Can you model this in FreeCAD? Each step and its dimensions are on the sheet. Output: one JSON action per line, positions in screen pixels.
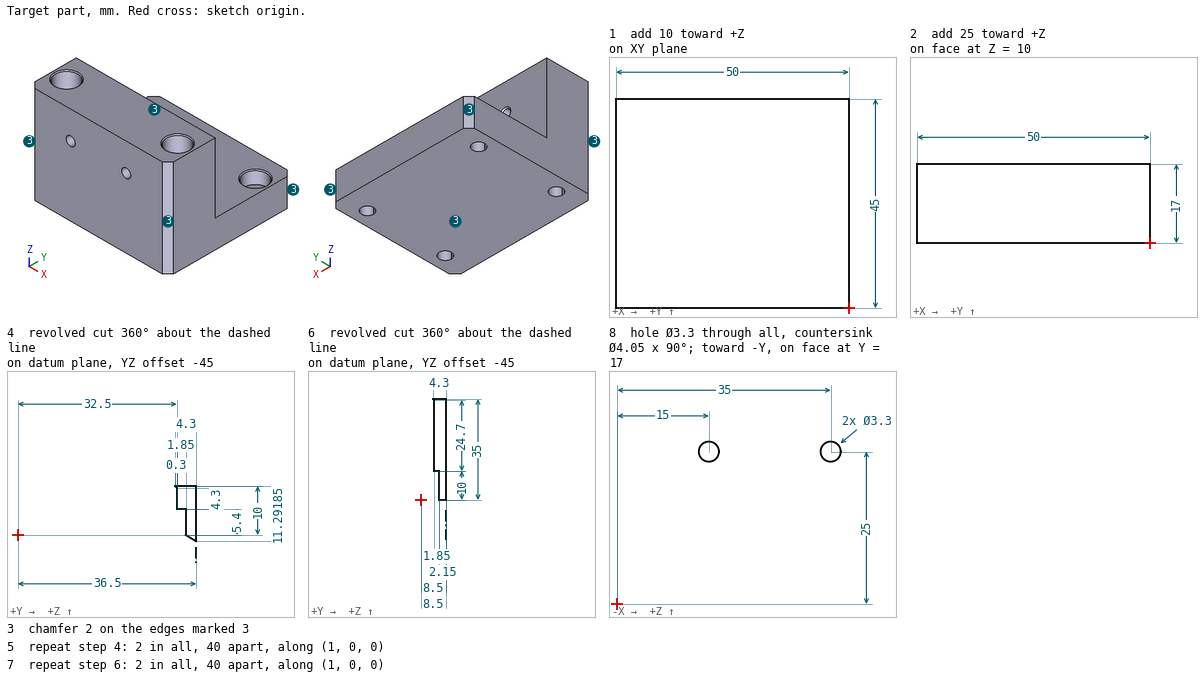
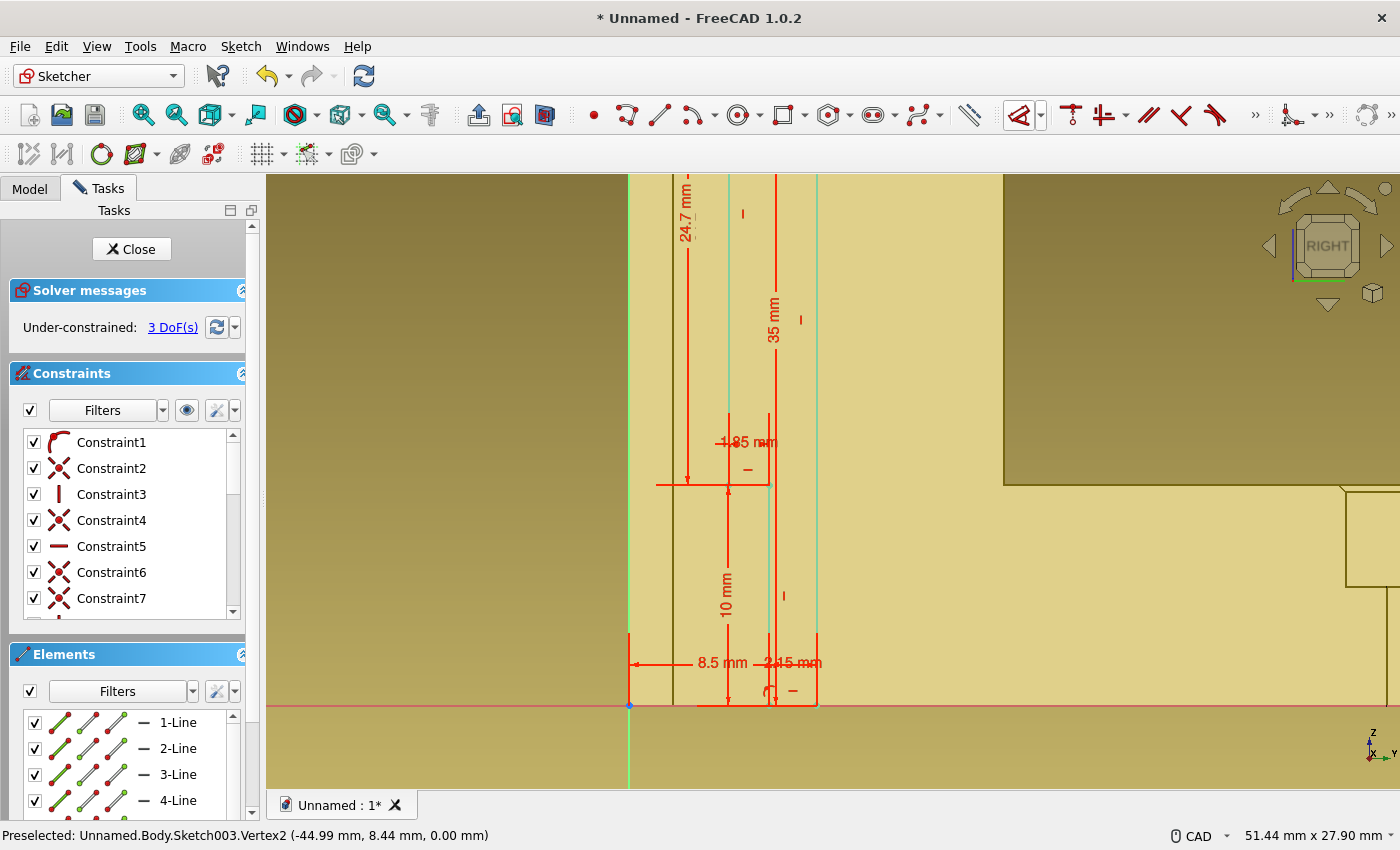
{"action": "scroll", "coordinate": [789, 486], "scroll_direction": "down", "scroll_amount": 5}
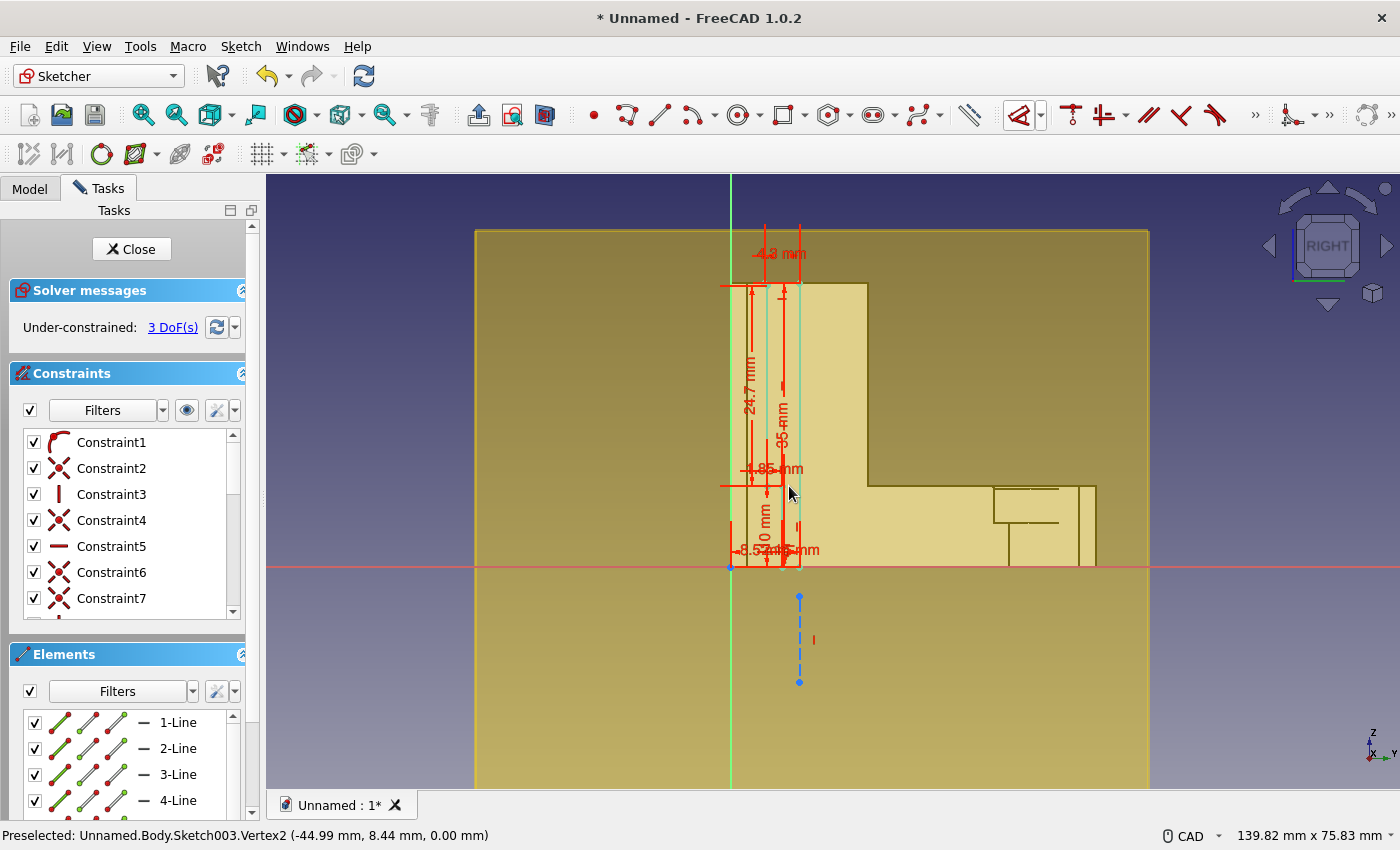
{"action": "left_click", "coordinate": [800, 596]}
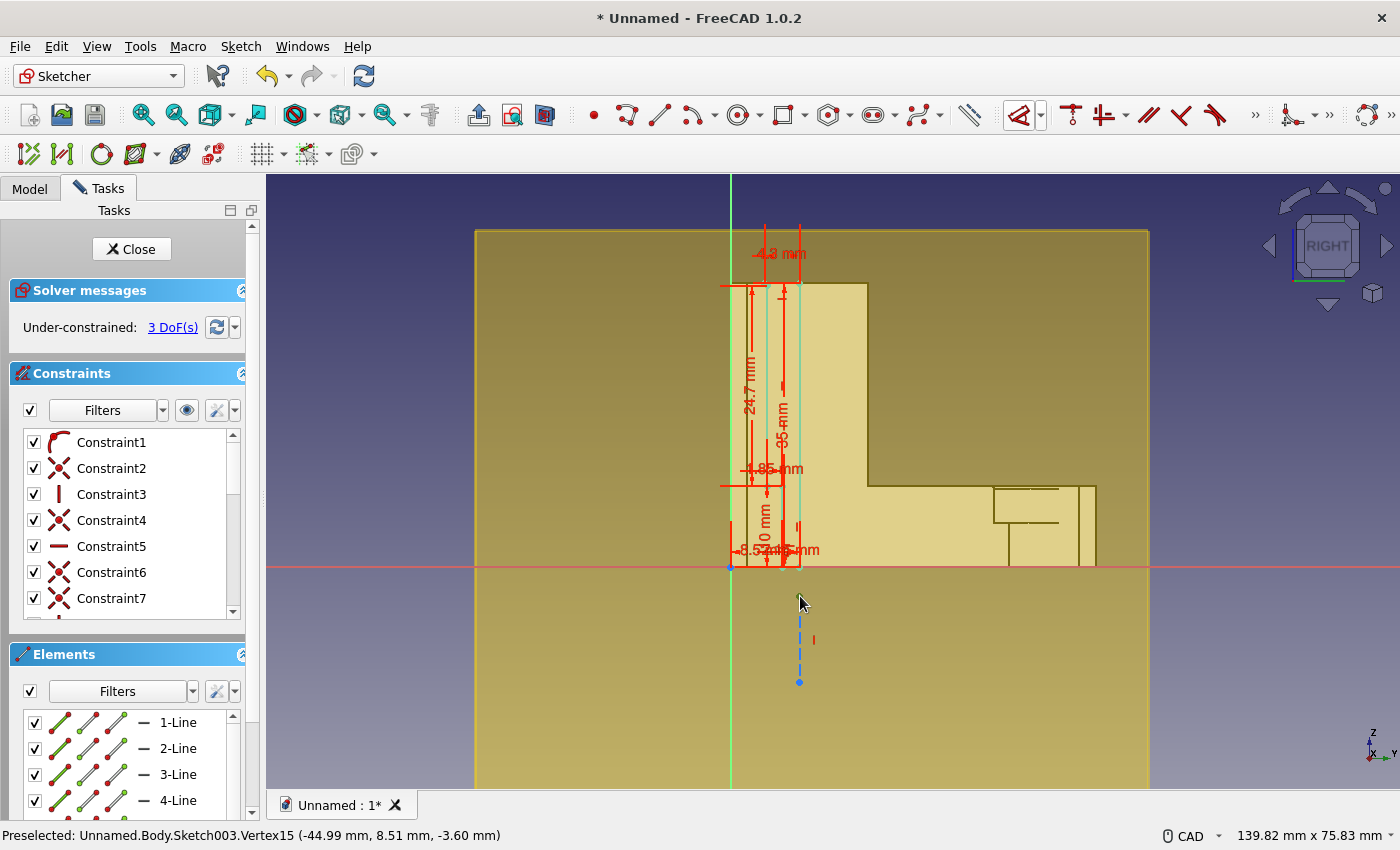
{"action": "left_click", "coordinate": [1040, 116]}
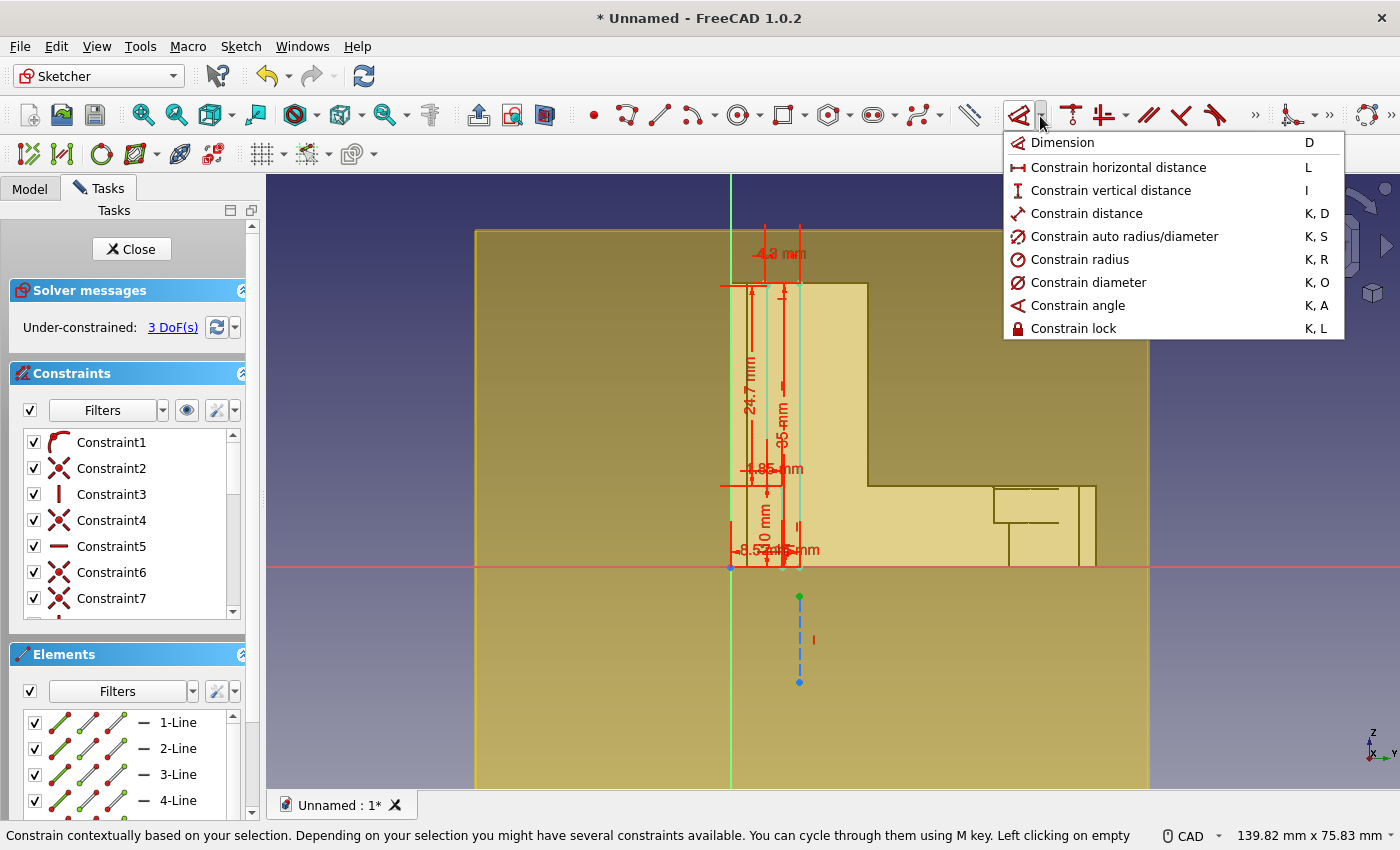
{"action": "left_click", "coordinate": [1174, 168]}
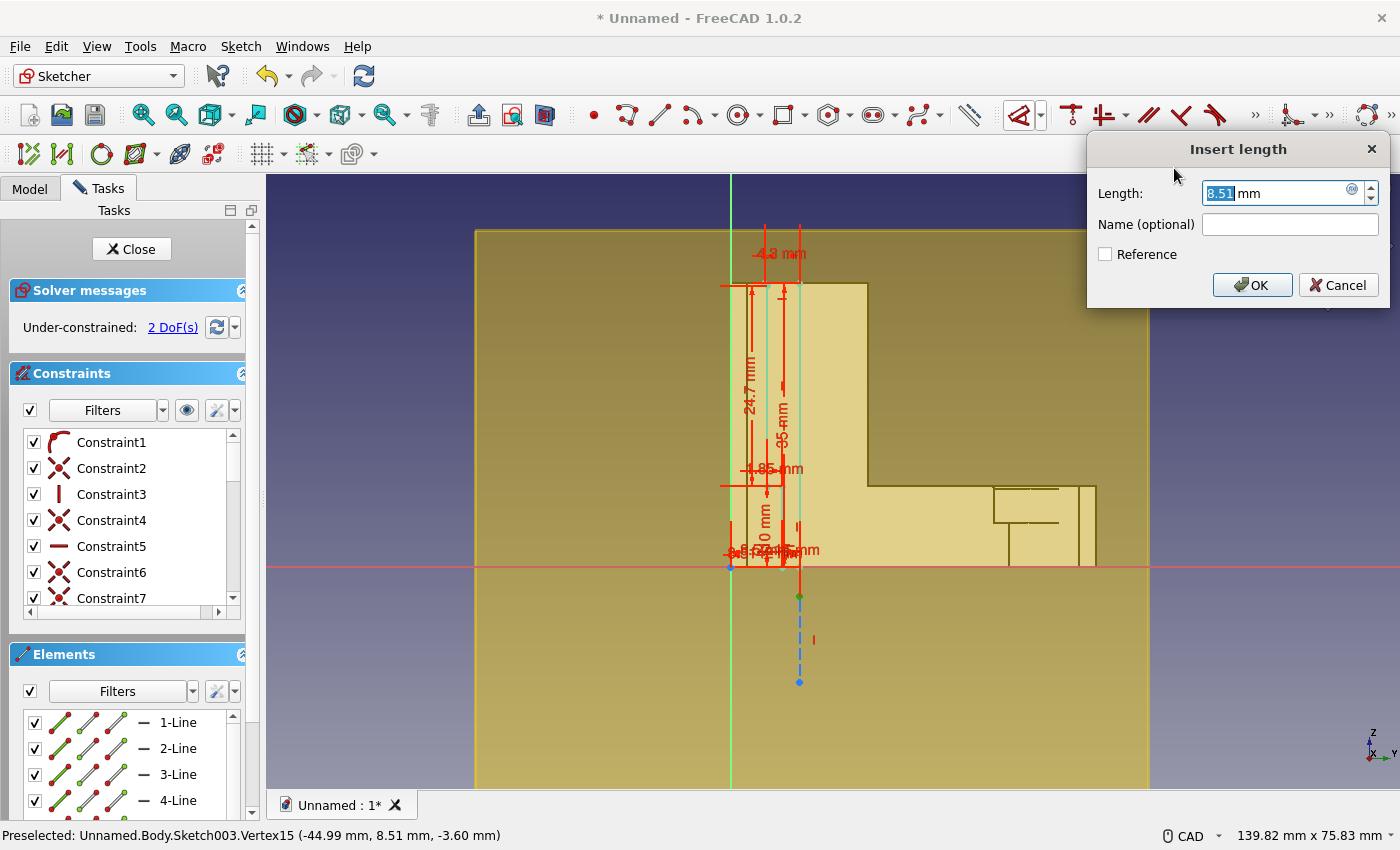
{"action": "type", "text": "8.5"}
{"action": "key", "text": "Return"}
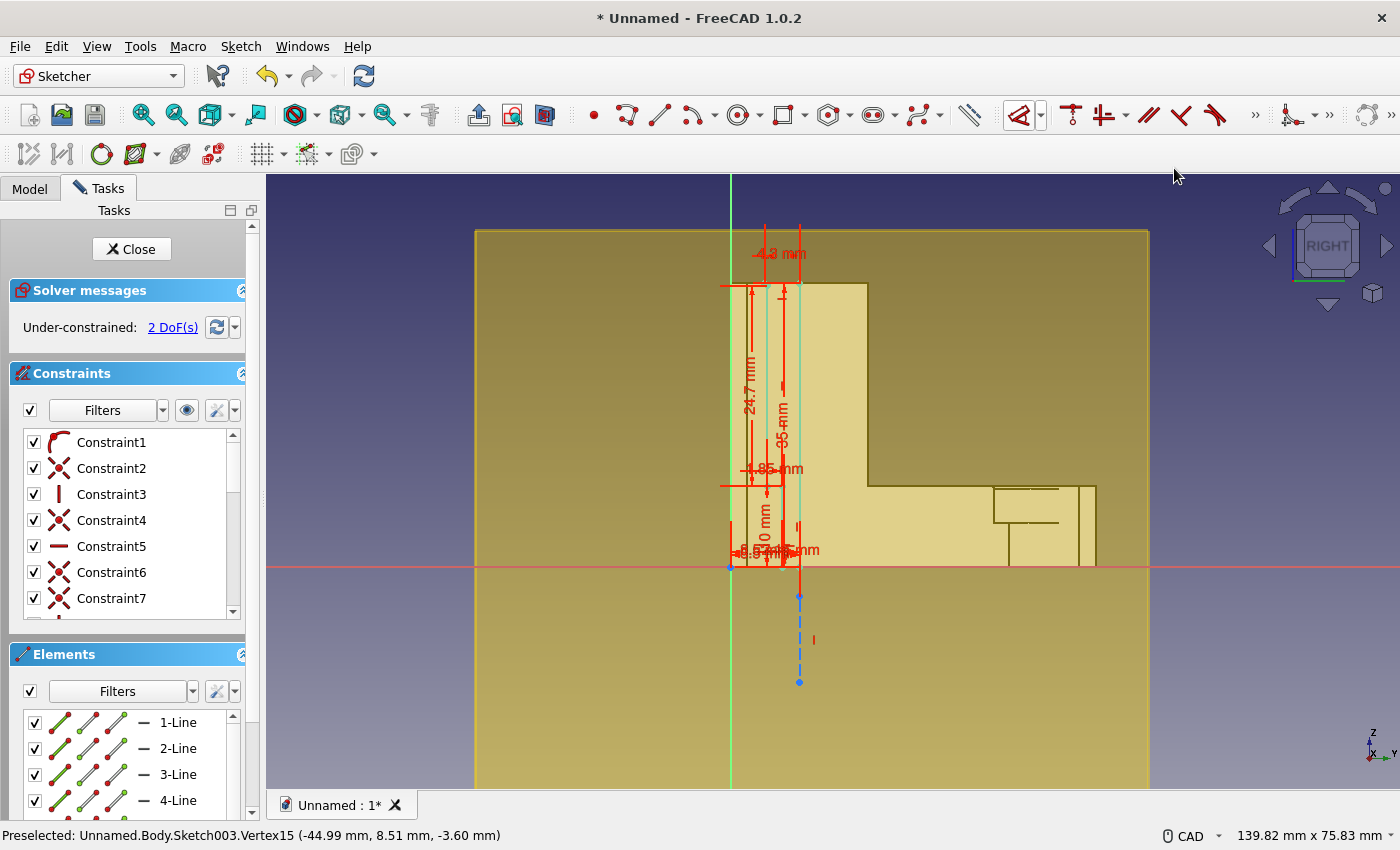
{"action": "left_click", "coordinate": [132, 249]}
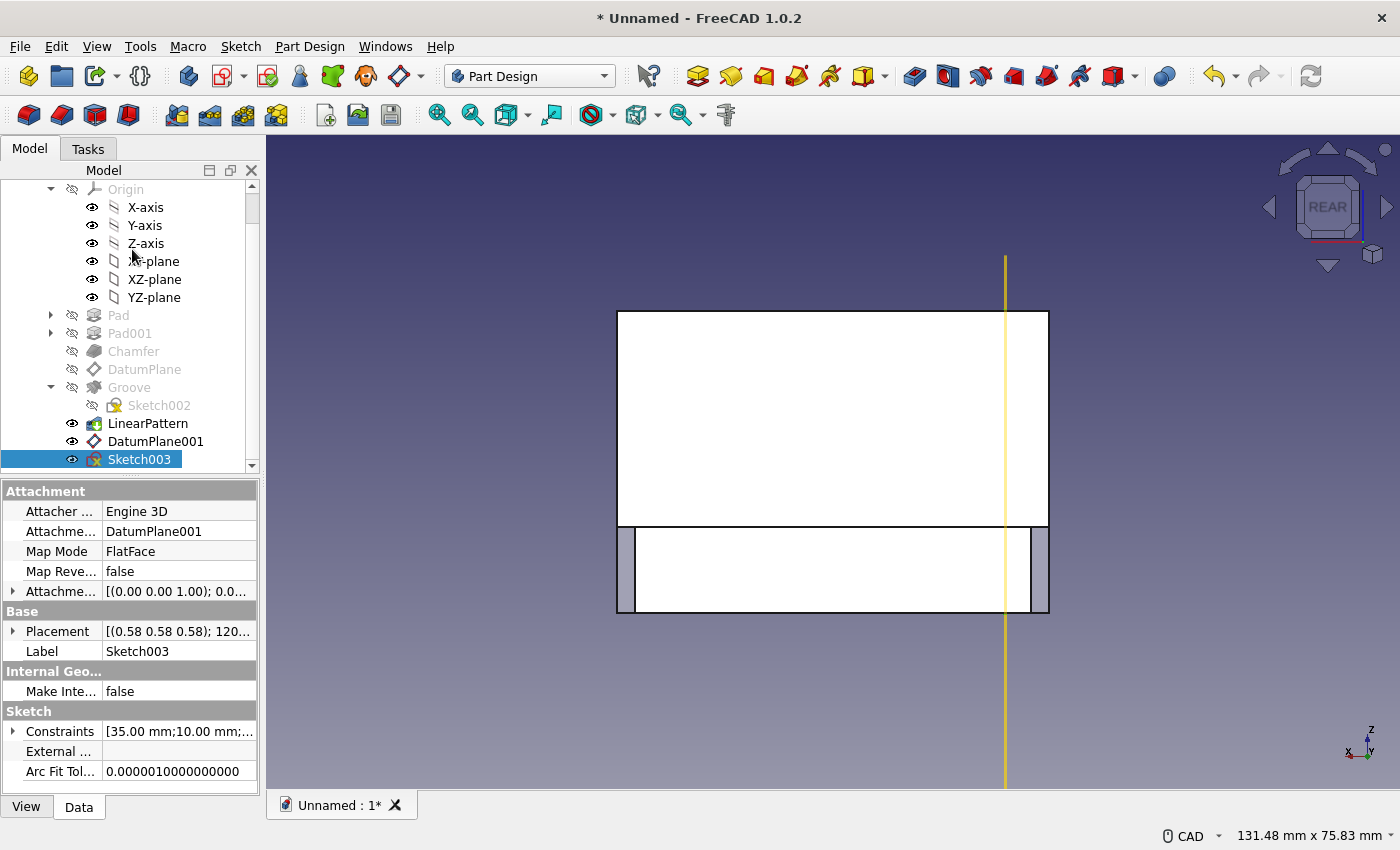
{"action": "left_click", "coordinate": [981, 76]}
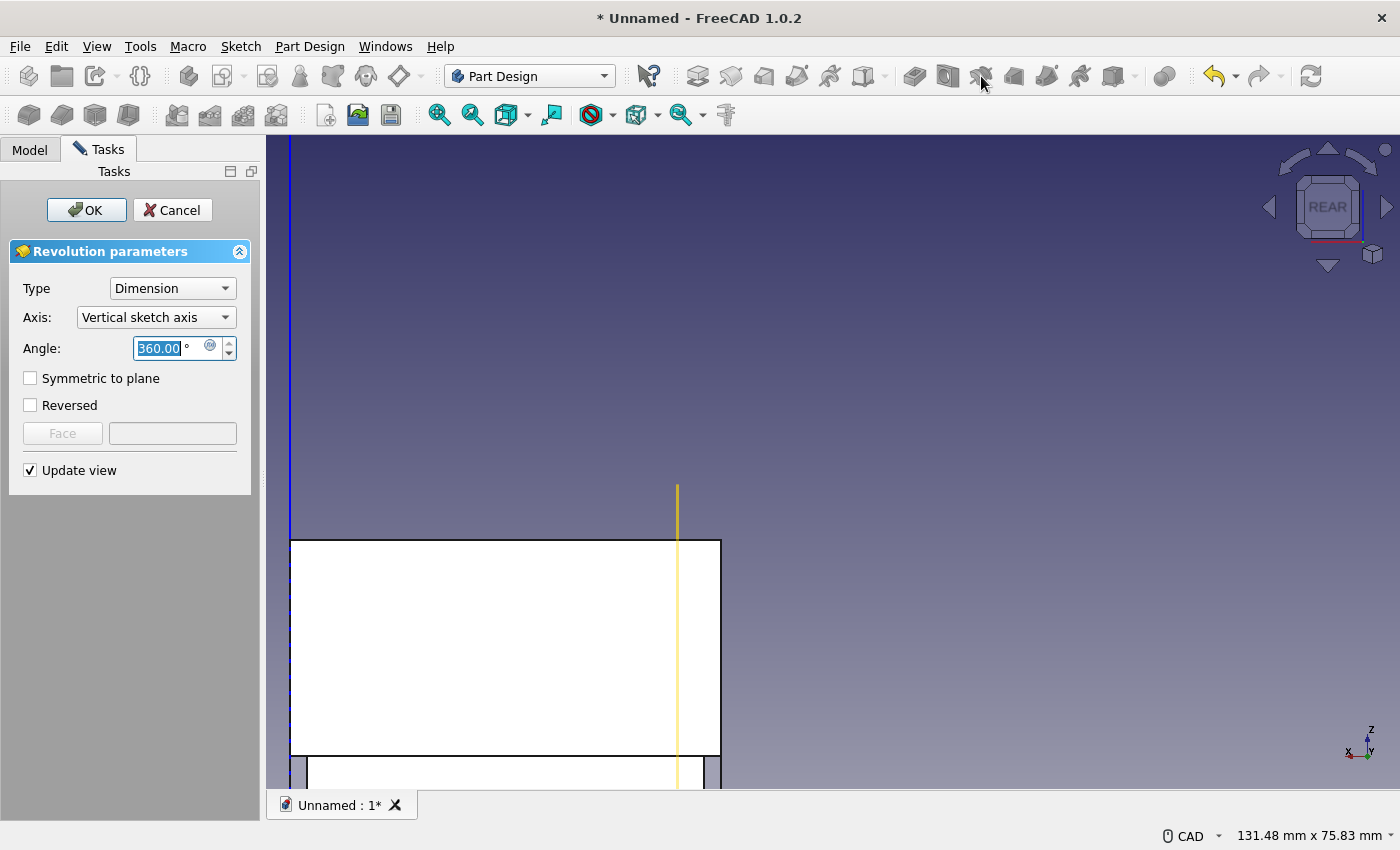
{"action": "left_click", "coordinate": [157, 318]}